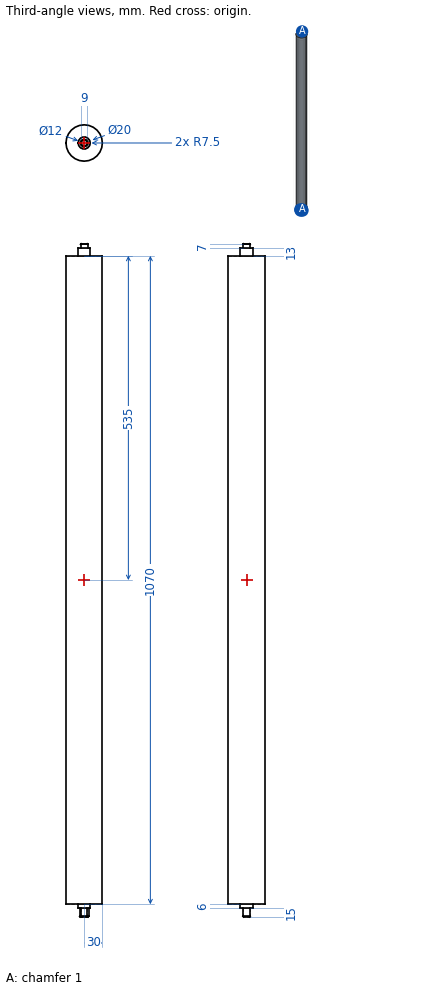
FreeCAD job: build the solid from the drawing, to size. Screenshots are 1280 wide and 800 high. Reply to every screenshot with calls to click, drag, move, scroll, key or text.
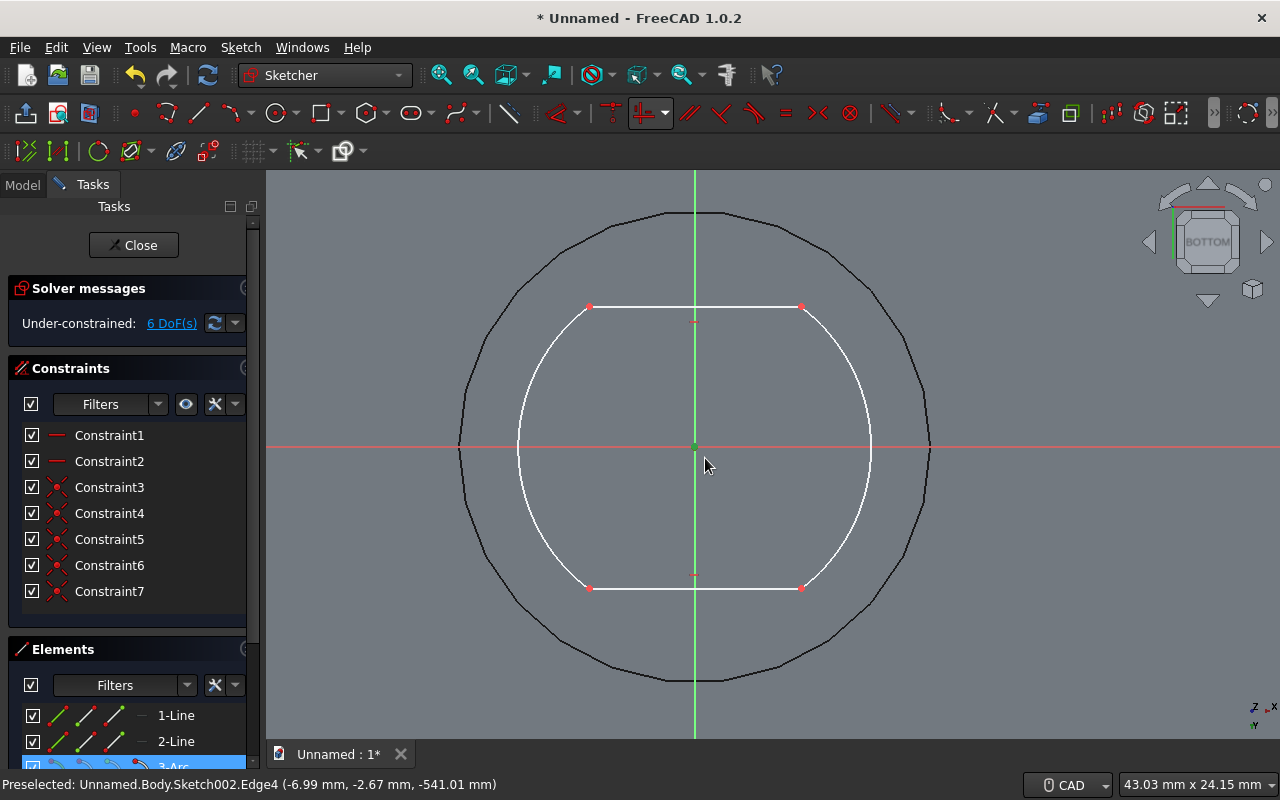
key(c)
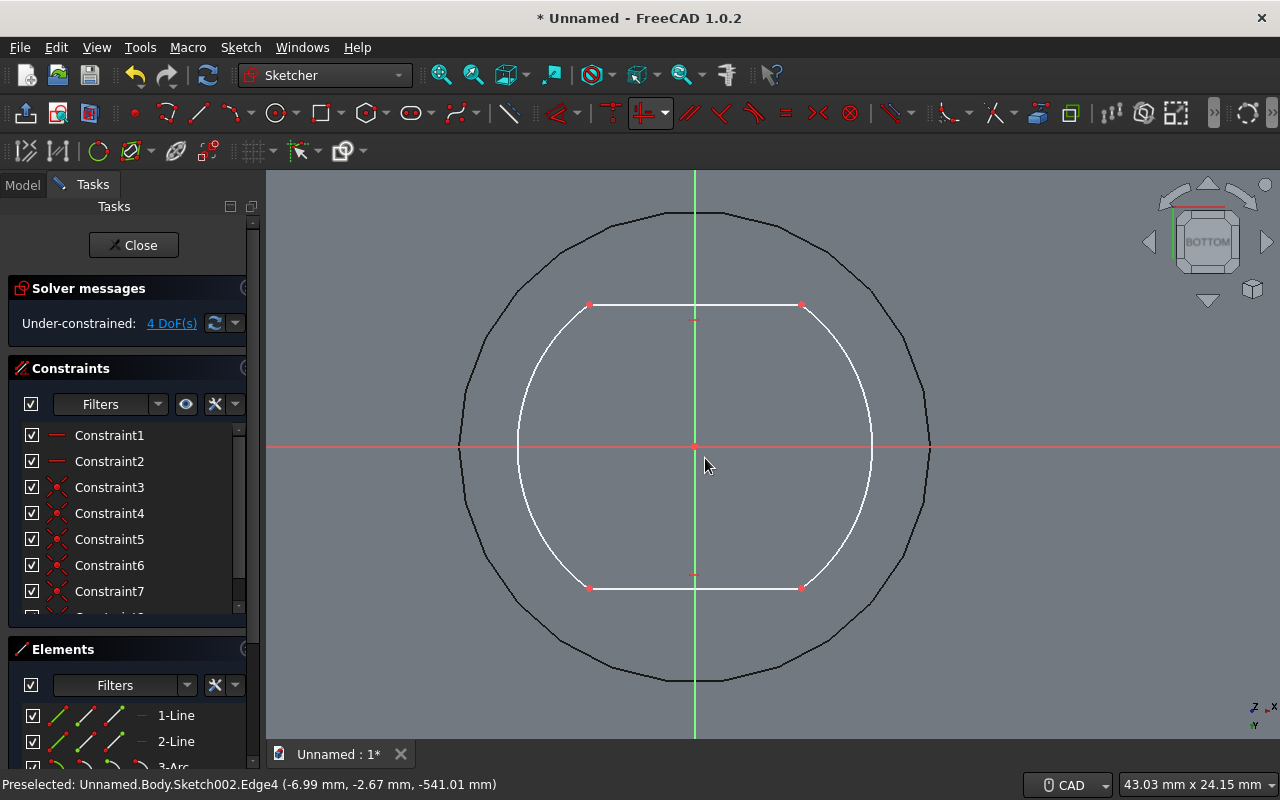
click(860, 511)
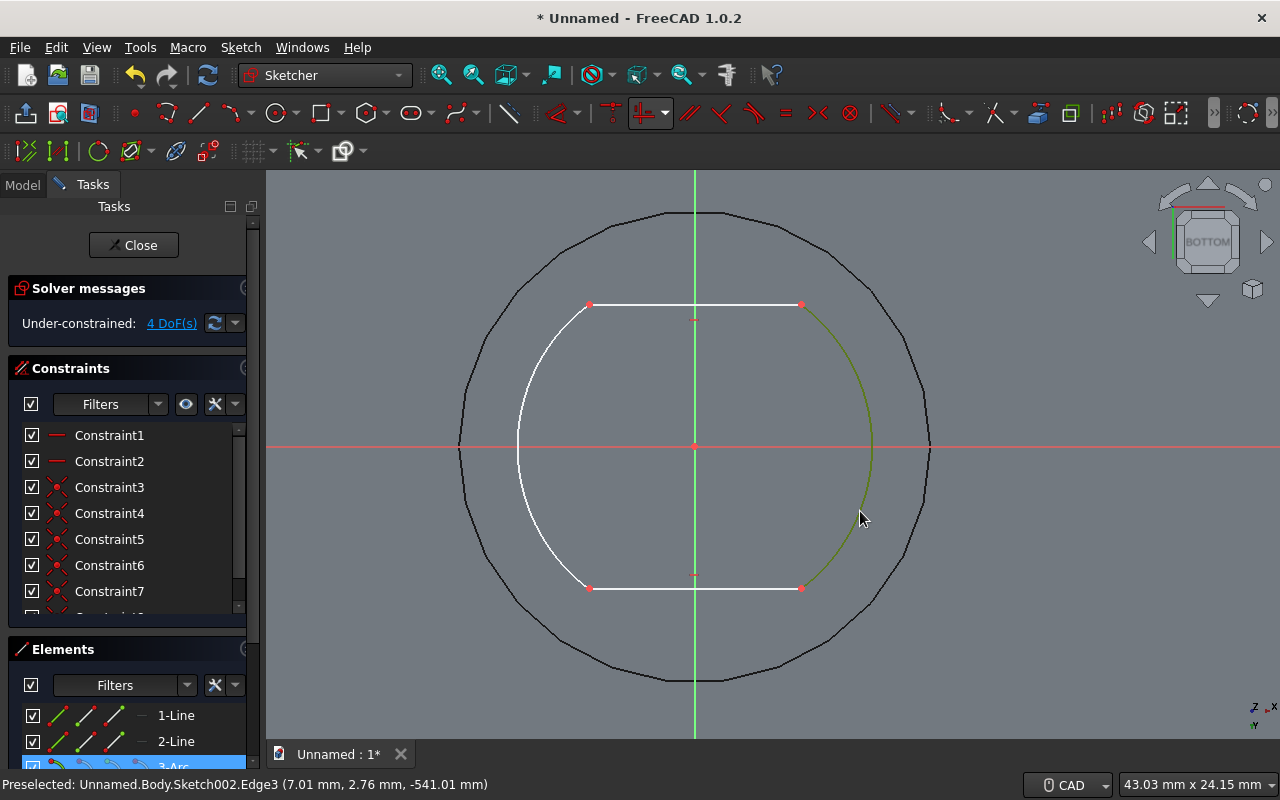
click(530, 382)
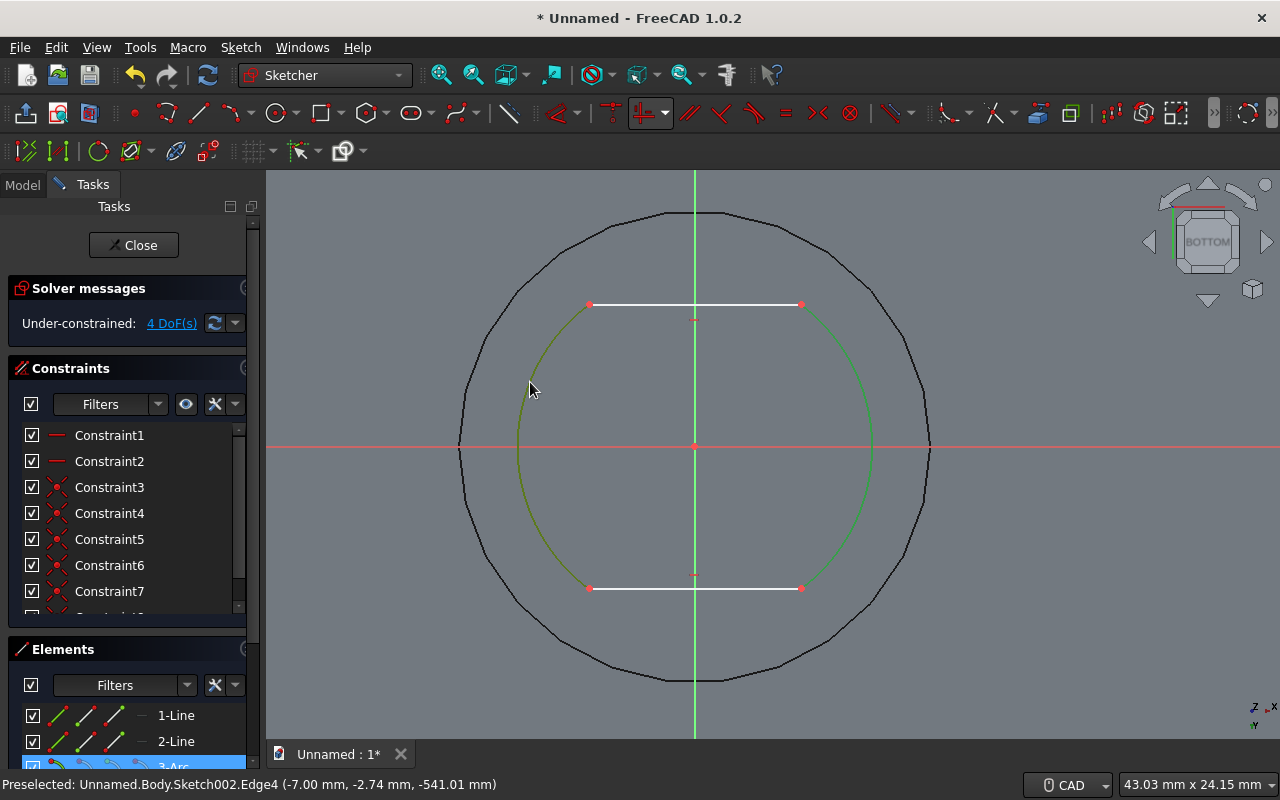
key(e)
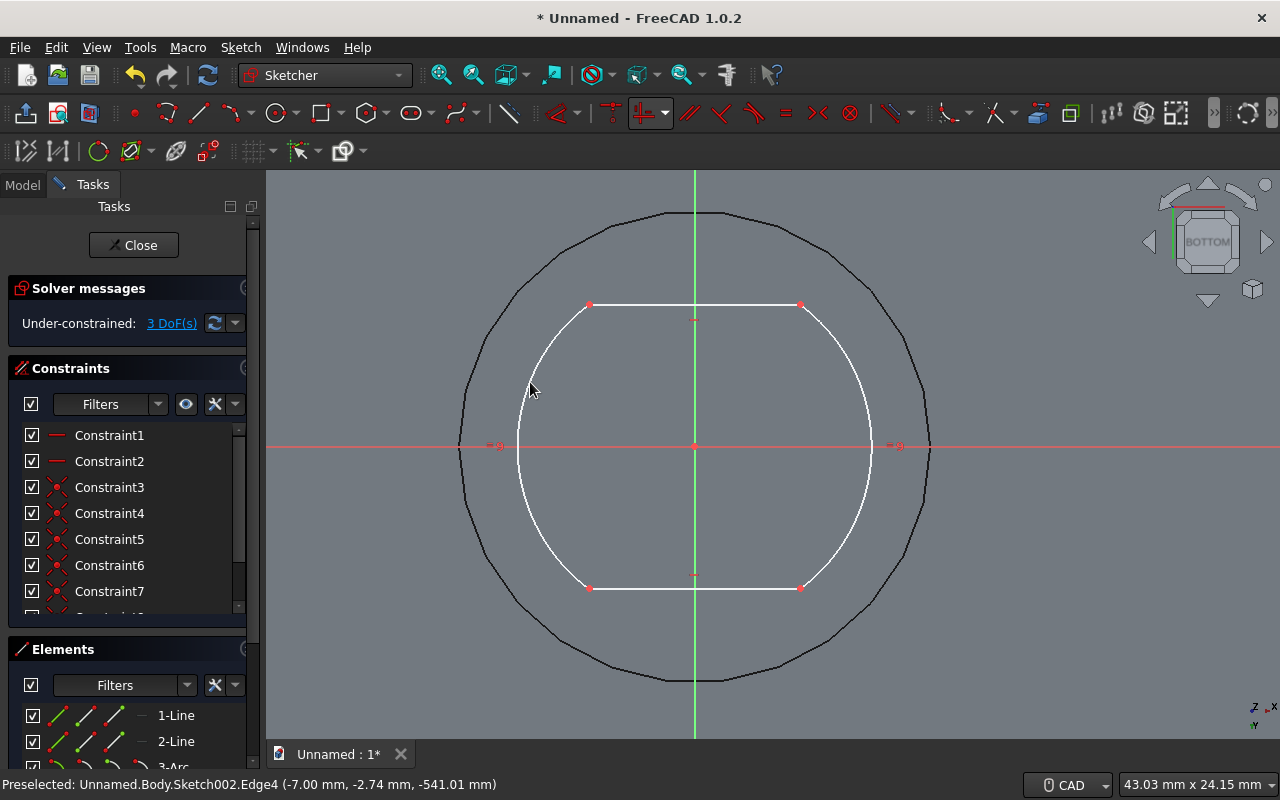
click(859, 511)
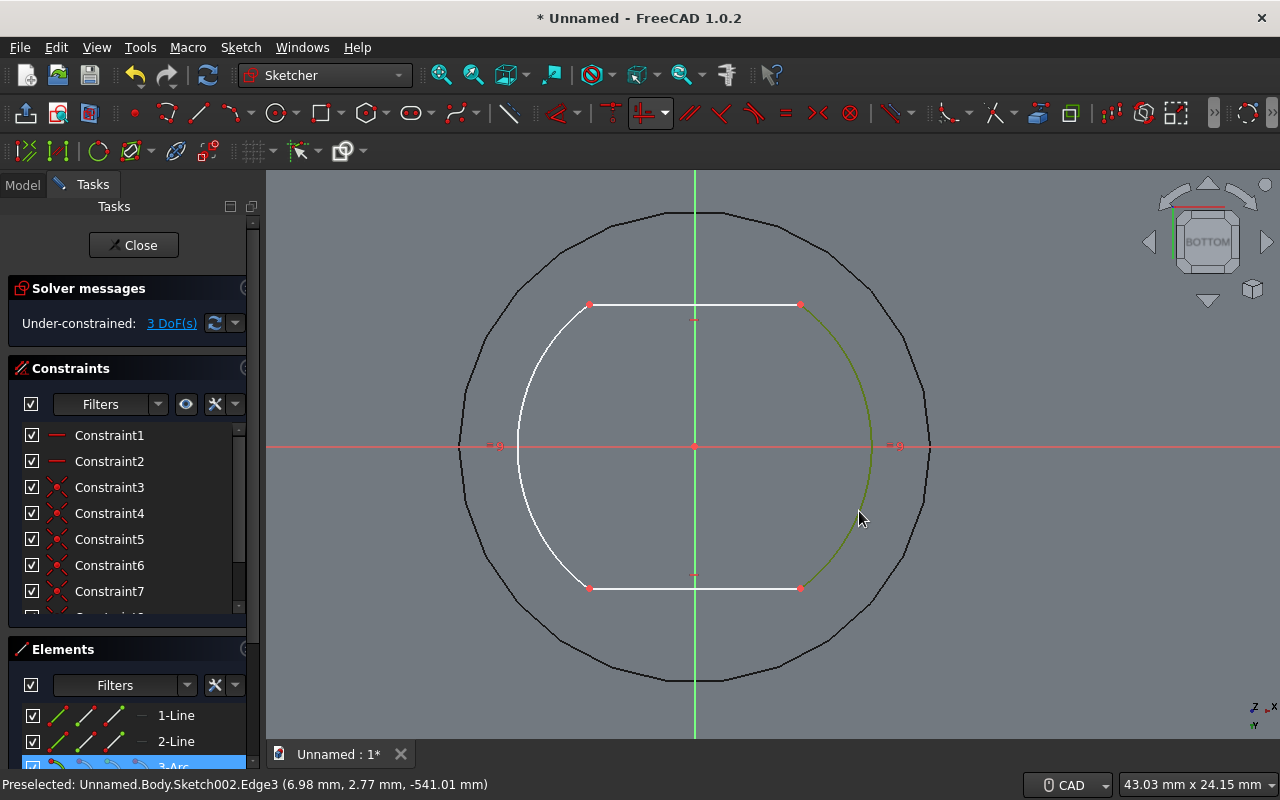
key(k)
key(r)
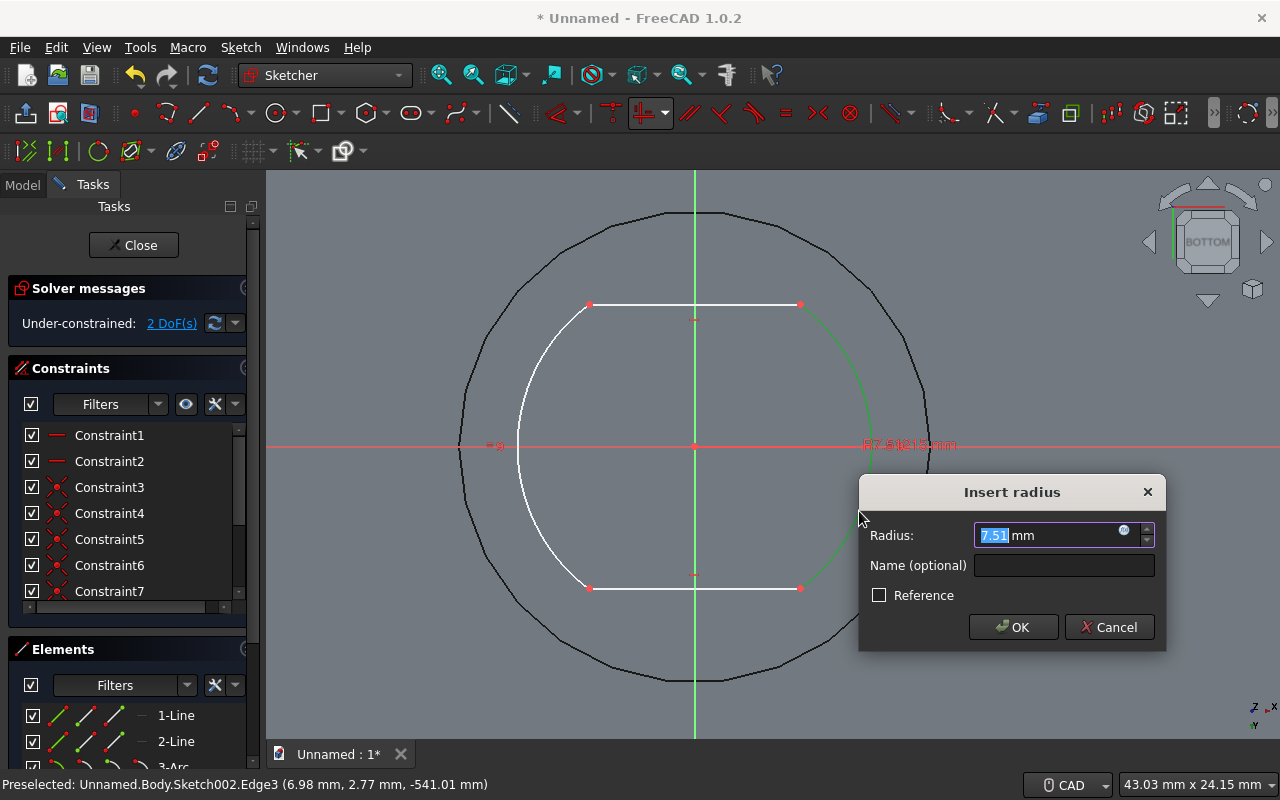
text(7.5)
key(Return)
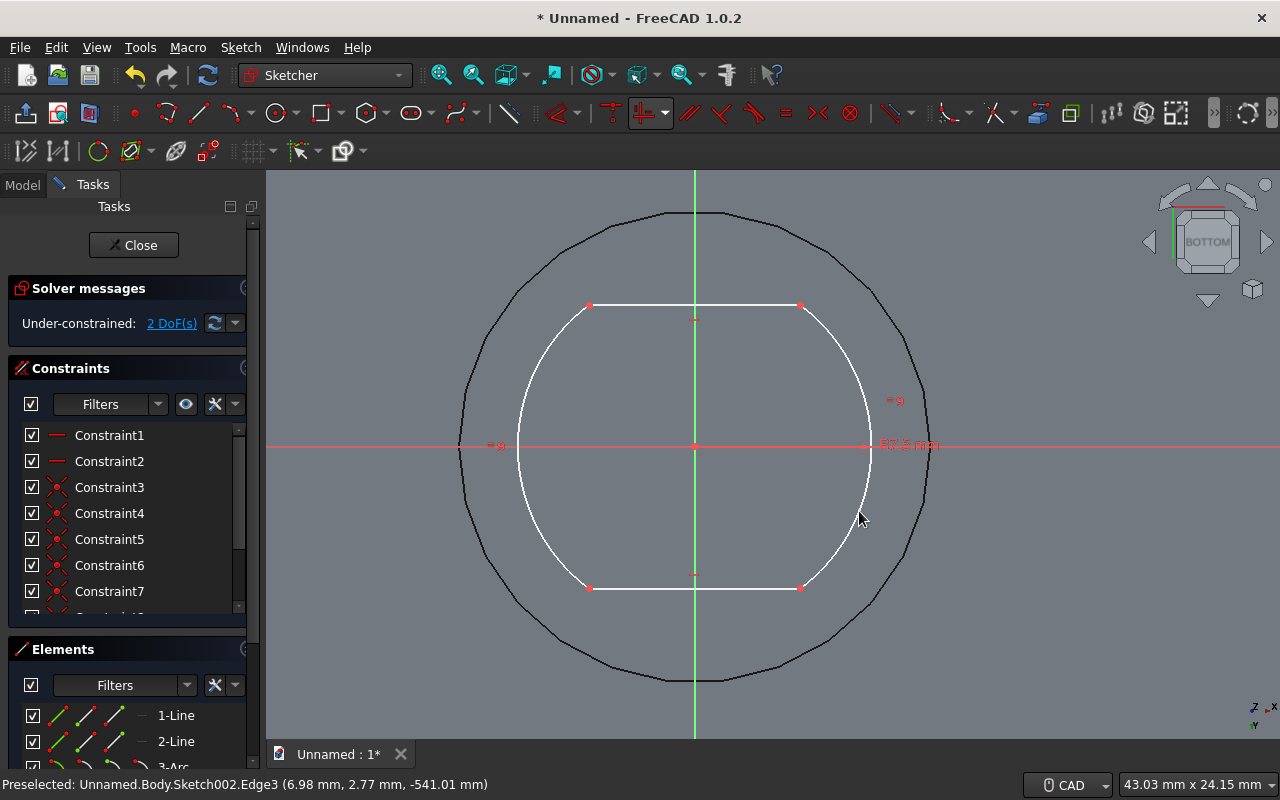
click(652, 589)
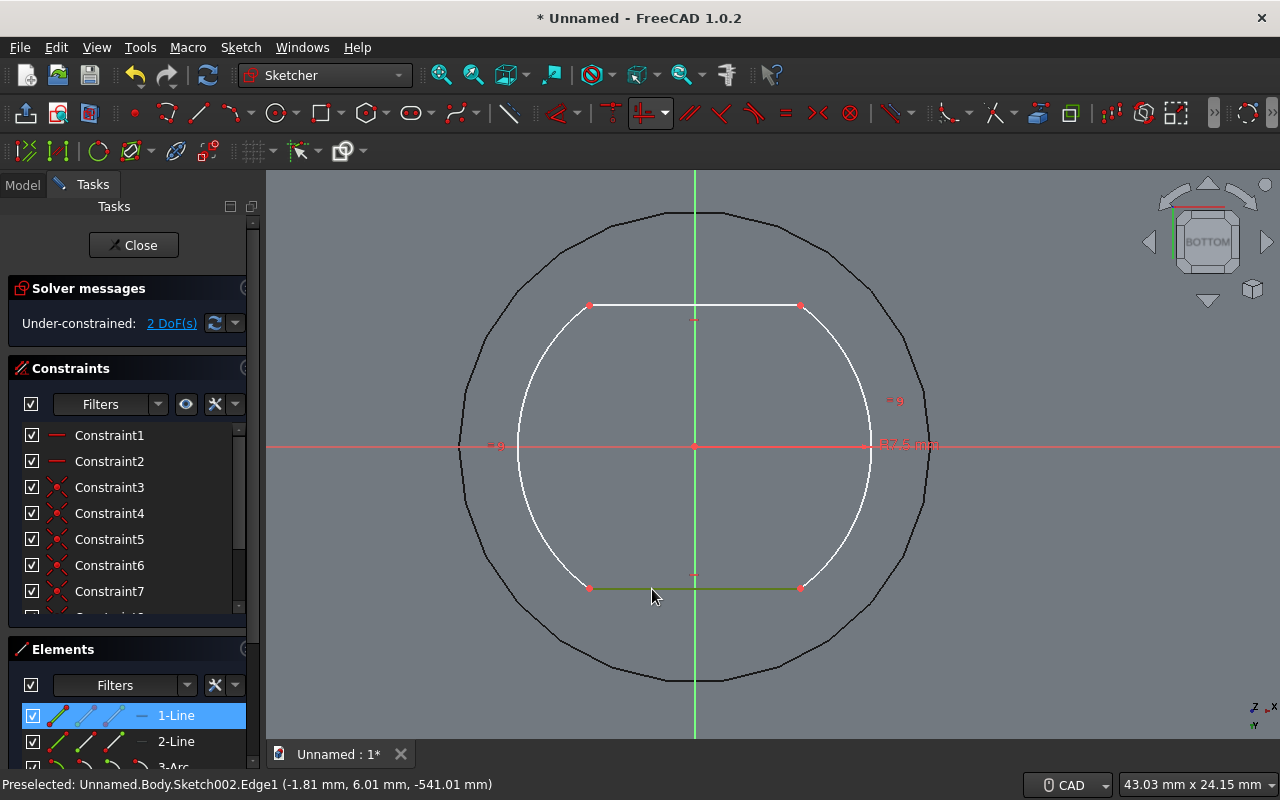
key(l)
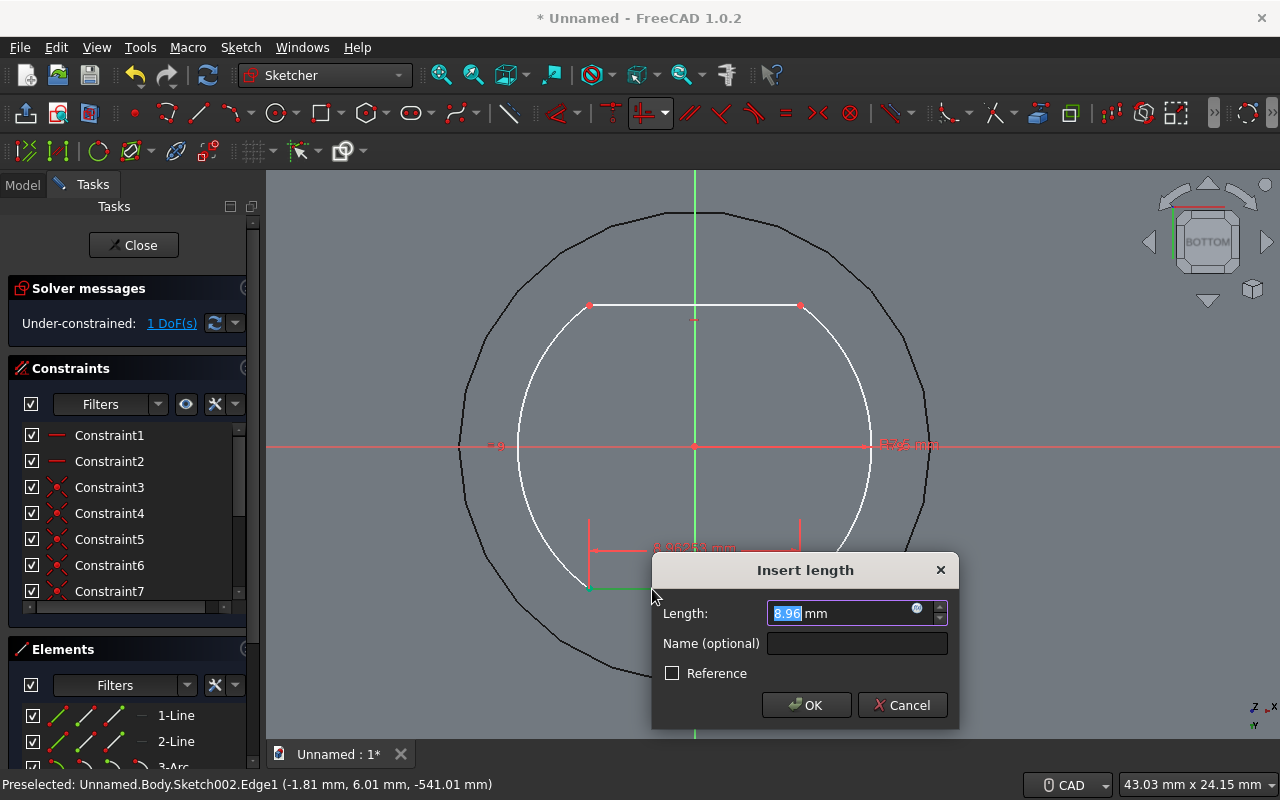
text(9)
key(Return)